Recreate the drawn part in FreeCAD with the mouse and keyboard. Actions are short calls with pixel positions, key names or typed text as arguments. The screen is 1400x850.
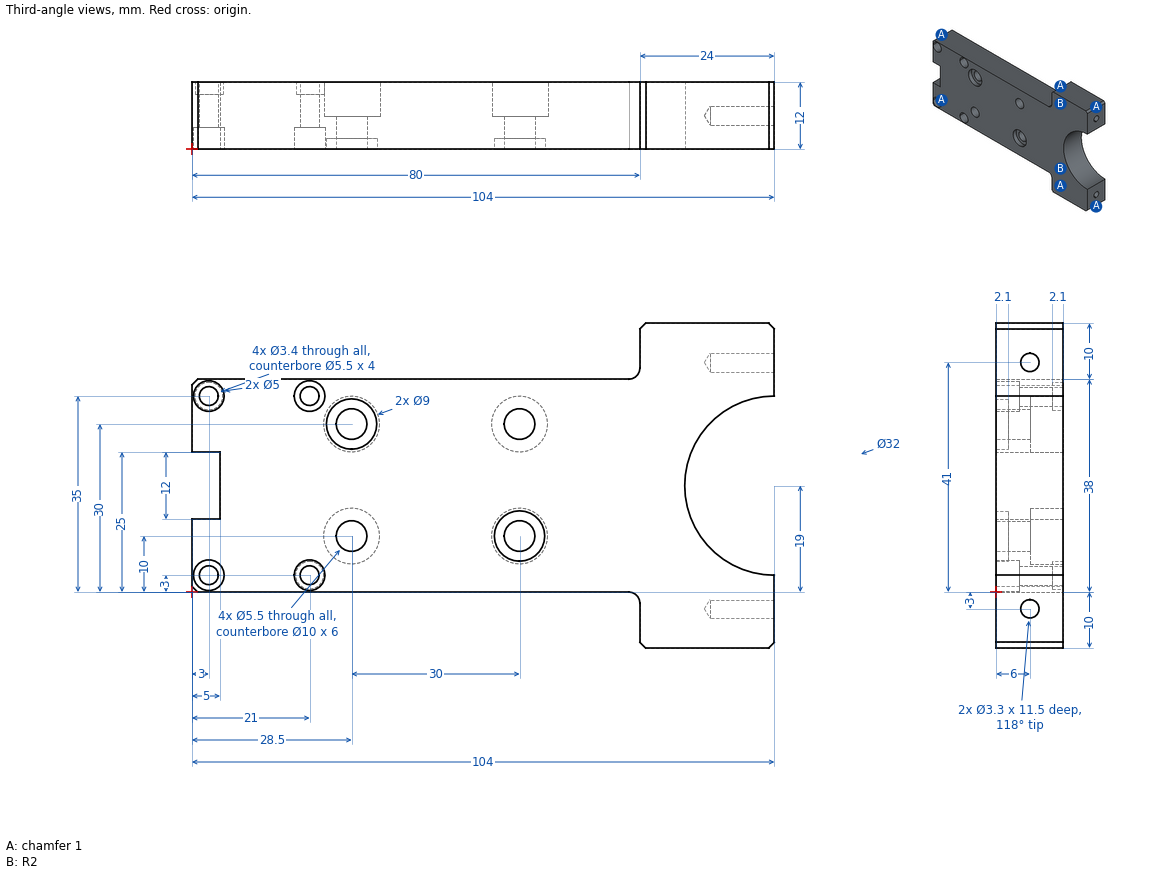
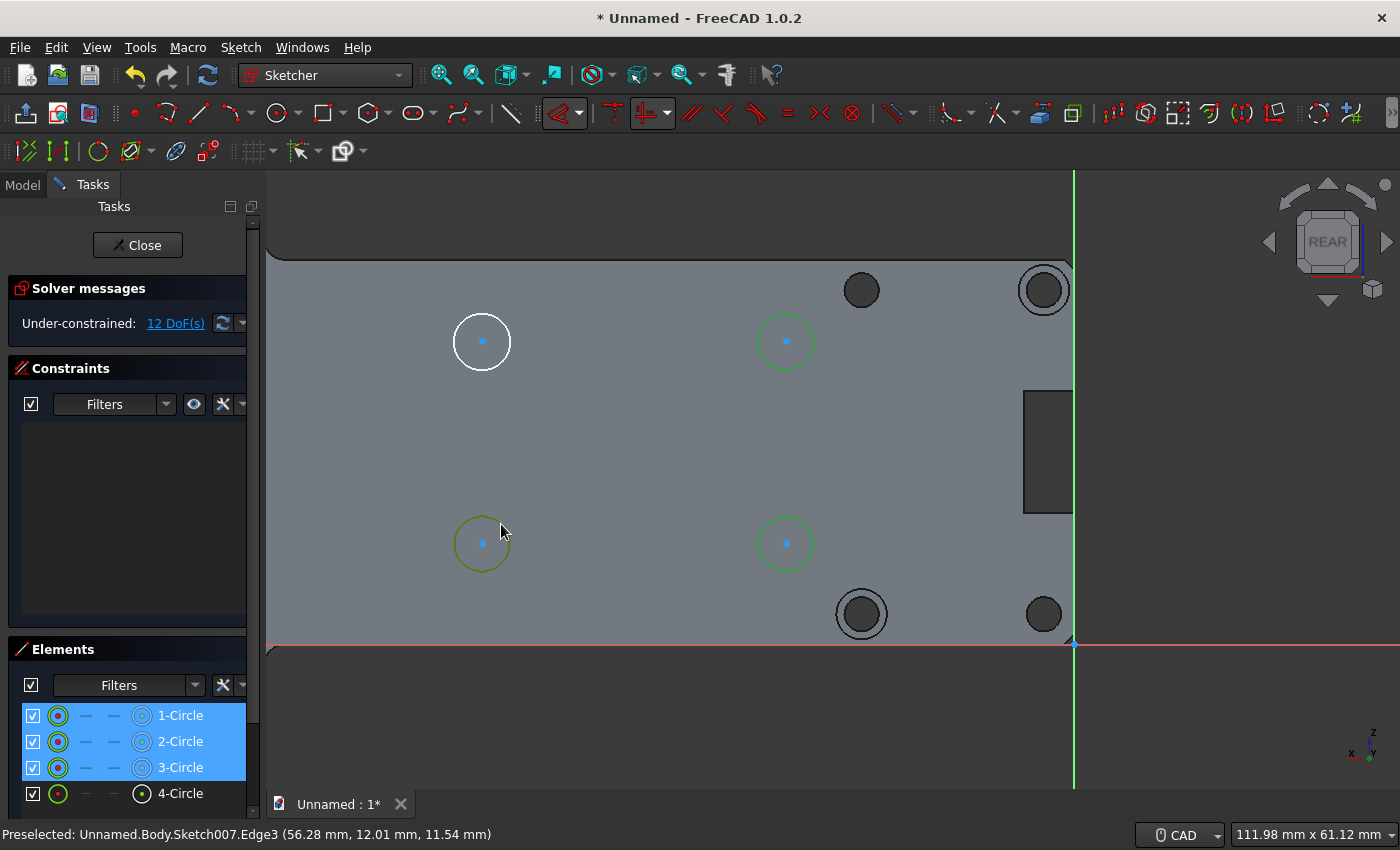
click(502, 322)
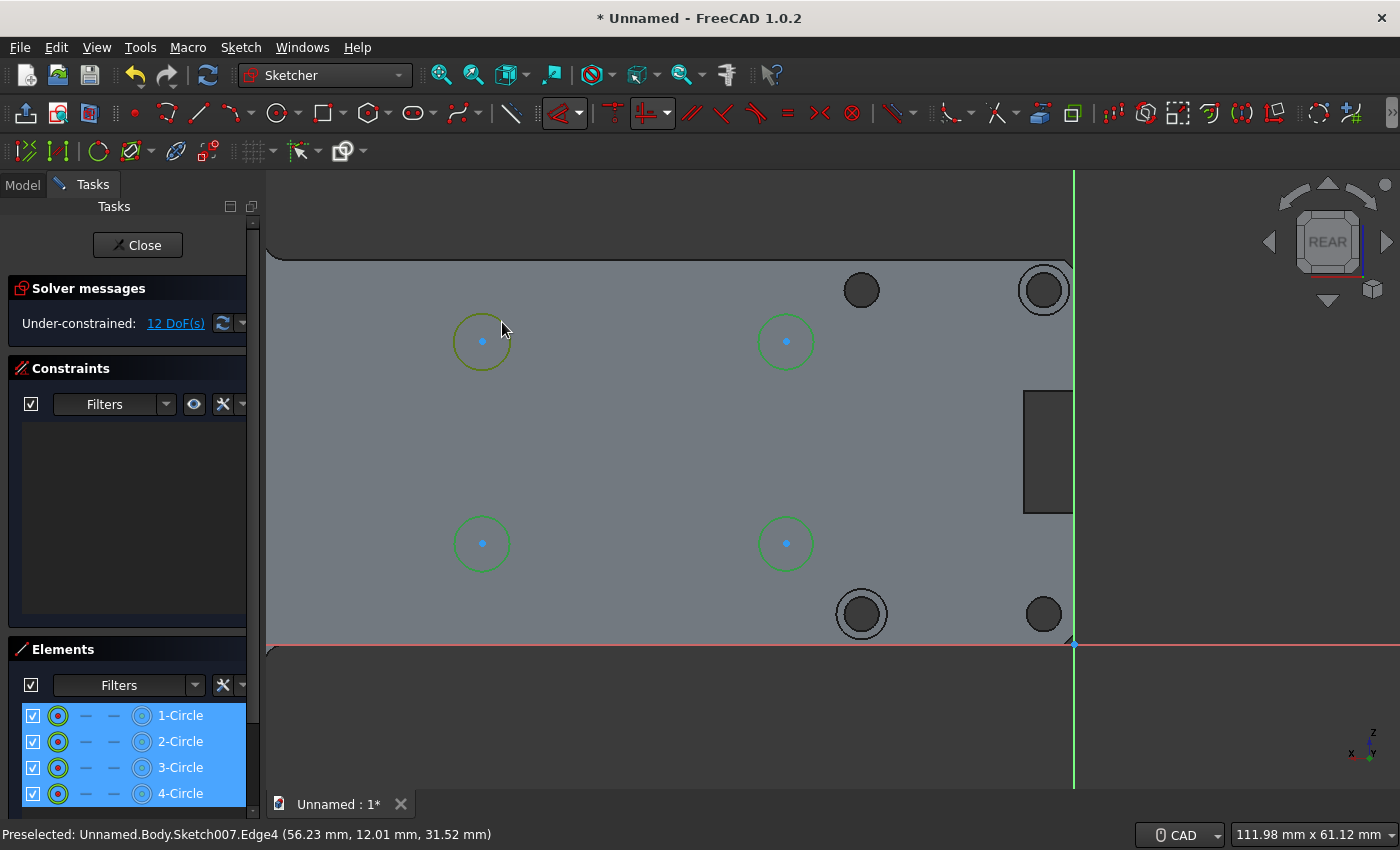
click(788, 114)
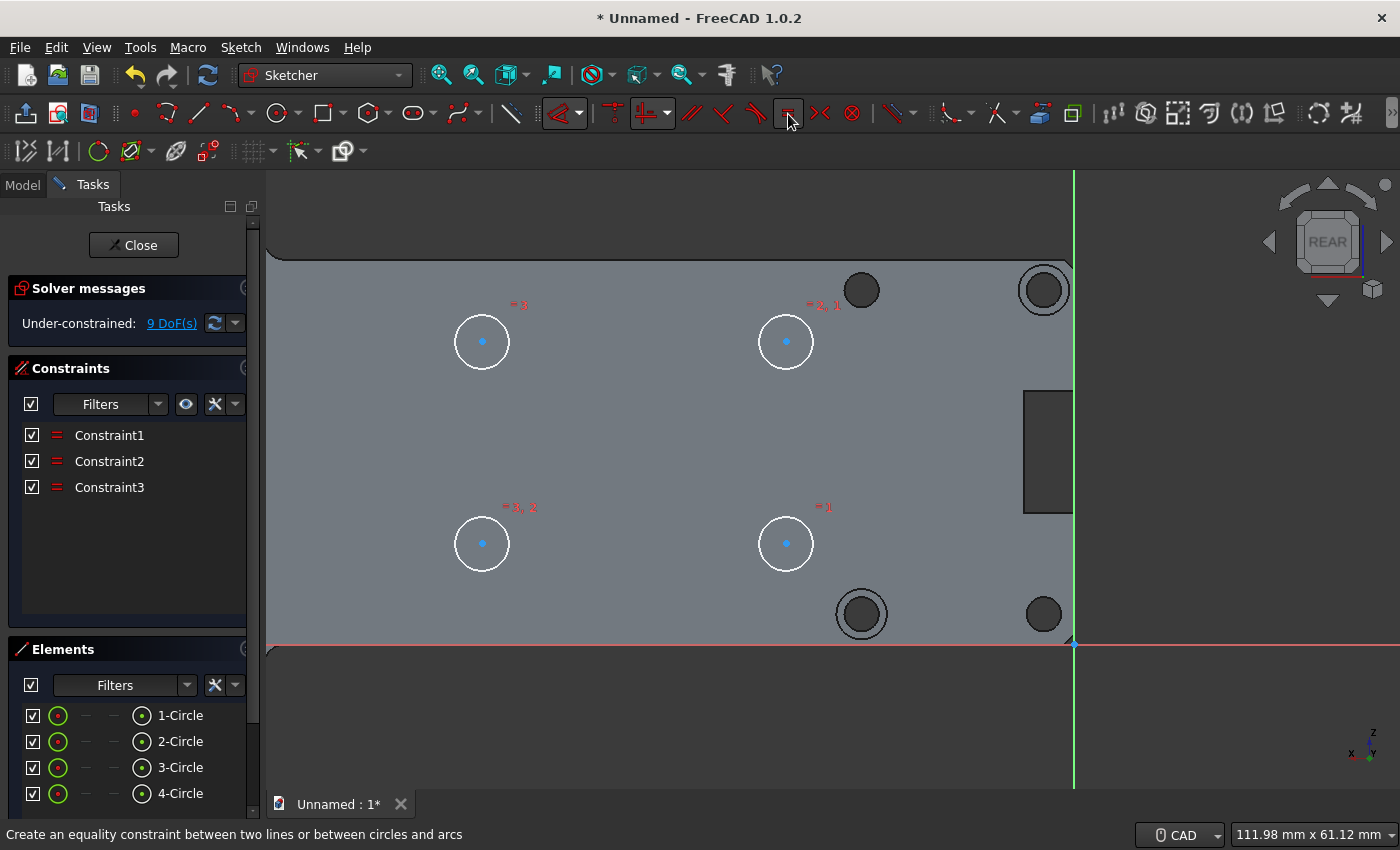
click(786, 544)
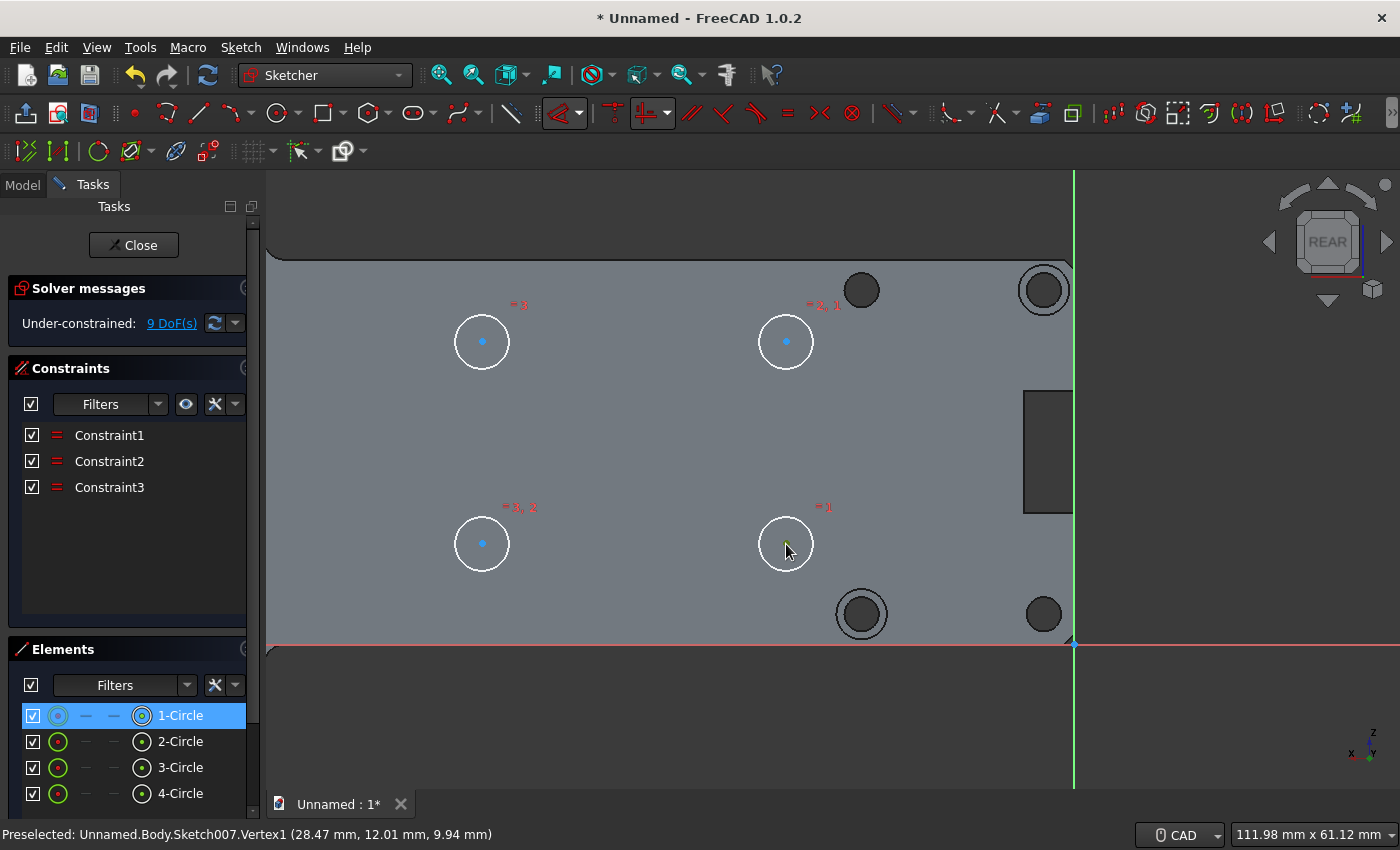
click(786, 342)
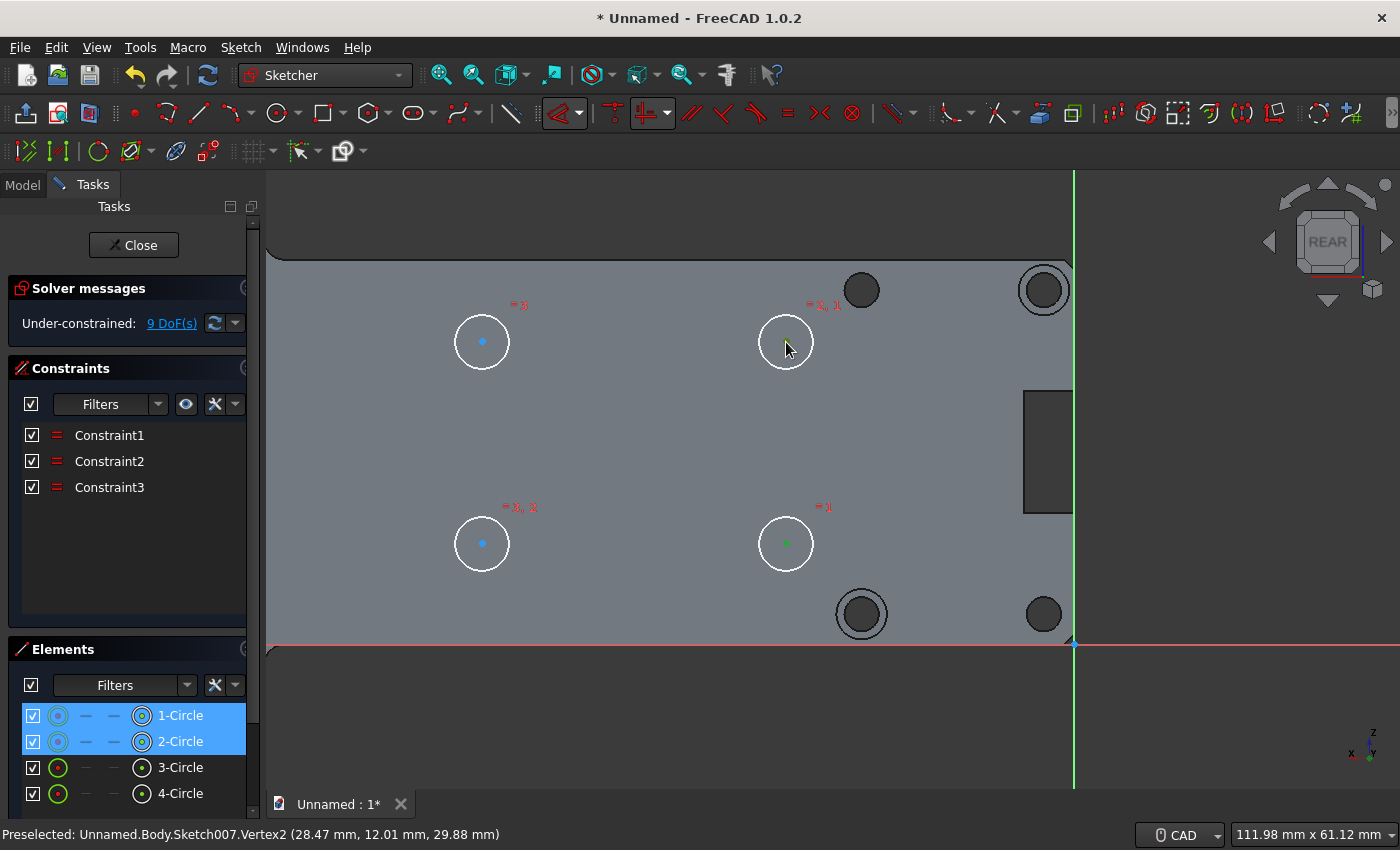
key(v)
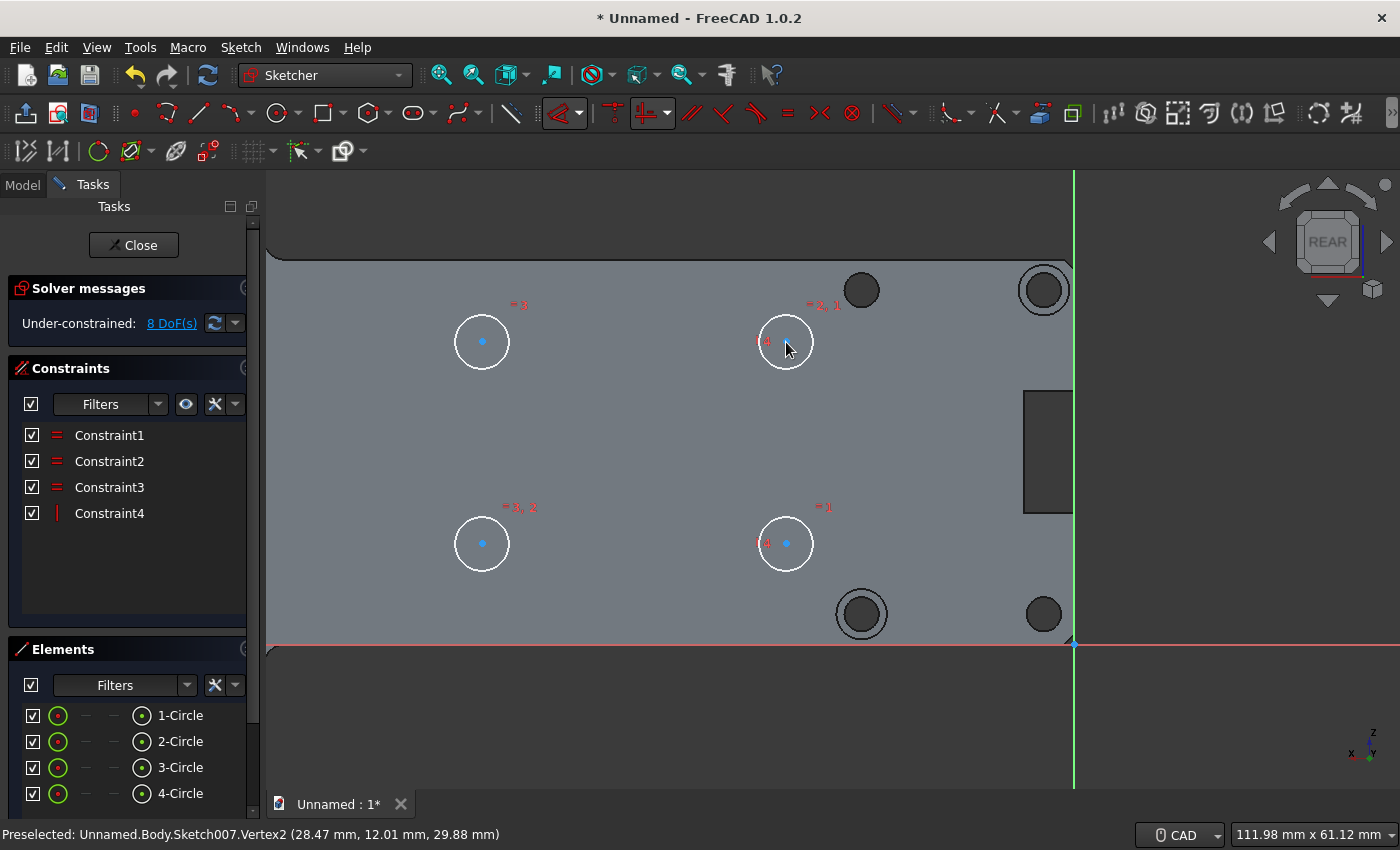
click(786, 544)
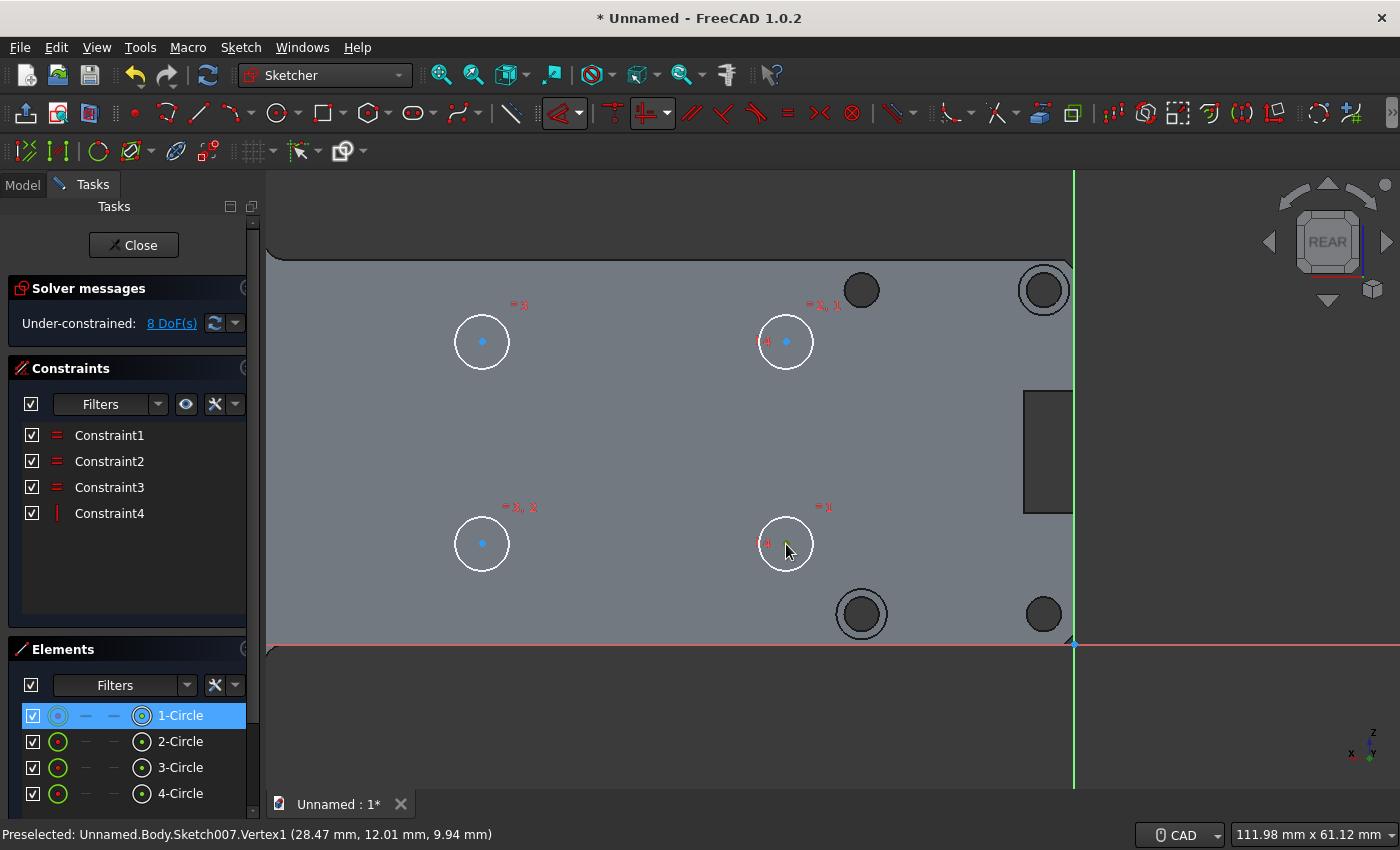
click(482, 544)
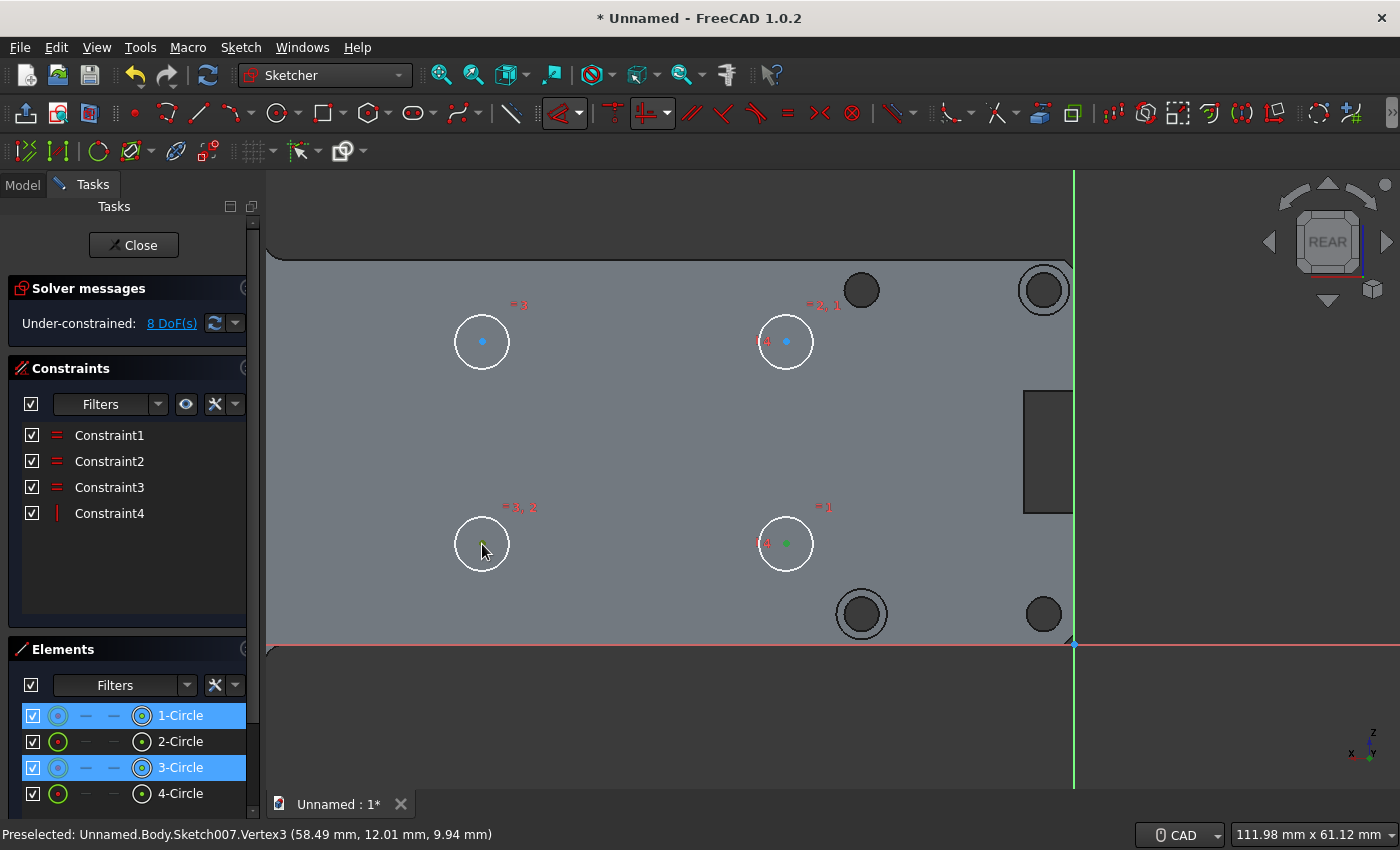
key(h)